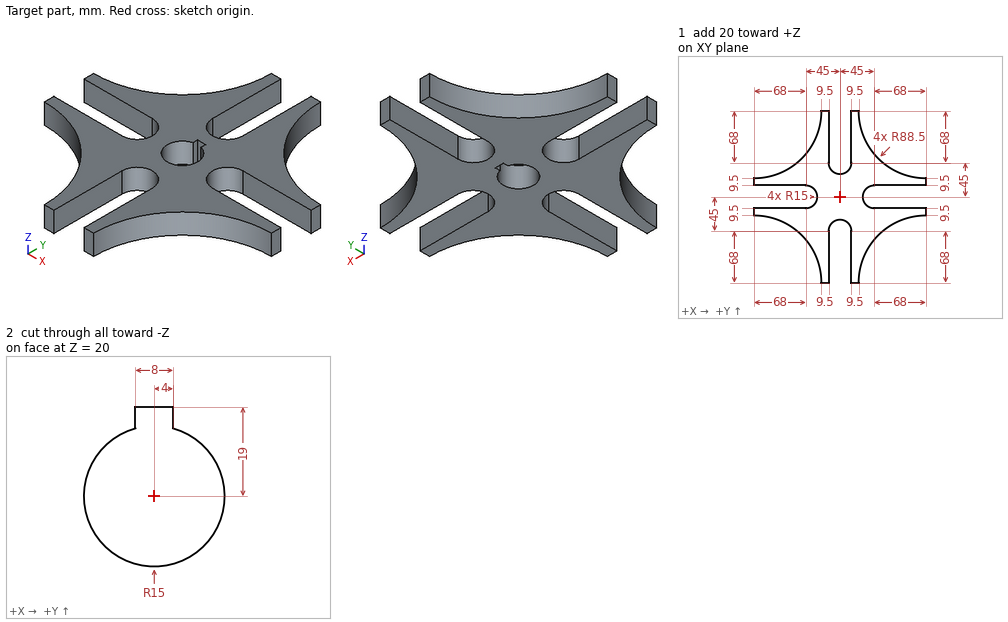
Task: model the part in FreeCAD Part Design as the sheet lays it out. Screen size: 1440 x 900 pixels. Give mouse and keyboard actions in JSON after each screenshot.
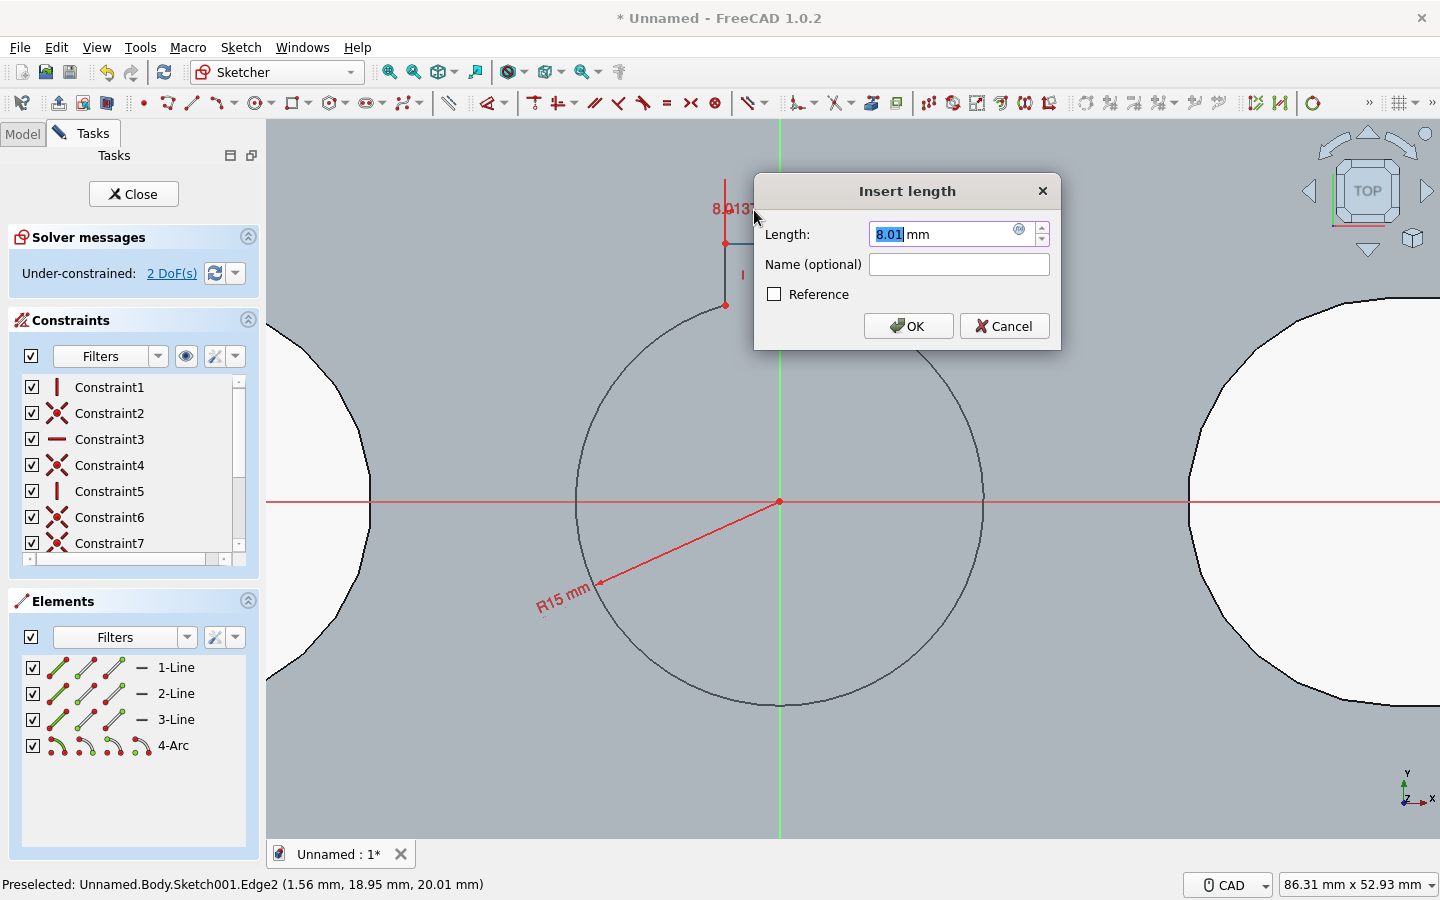
{"action": "type", "text": "8"}
{"action": "key", "text": "Return"}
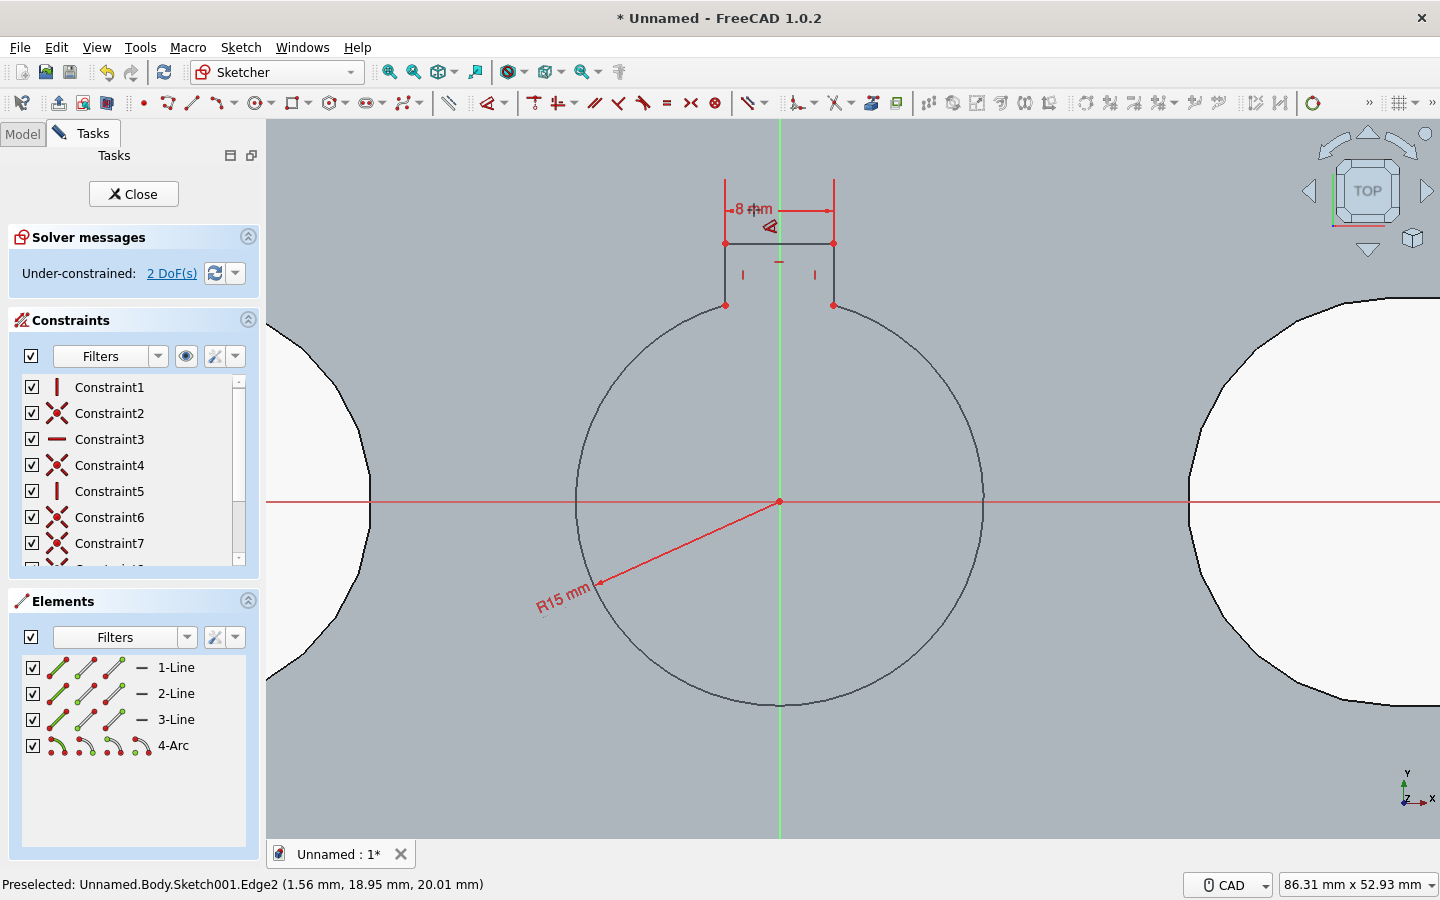
{"action": "left_click", "coordinate": [834, 305]}
{"action": "left_click", "coordinate": [807, 271]}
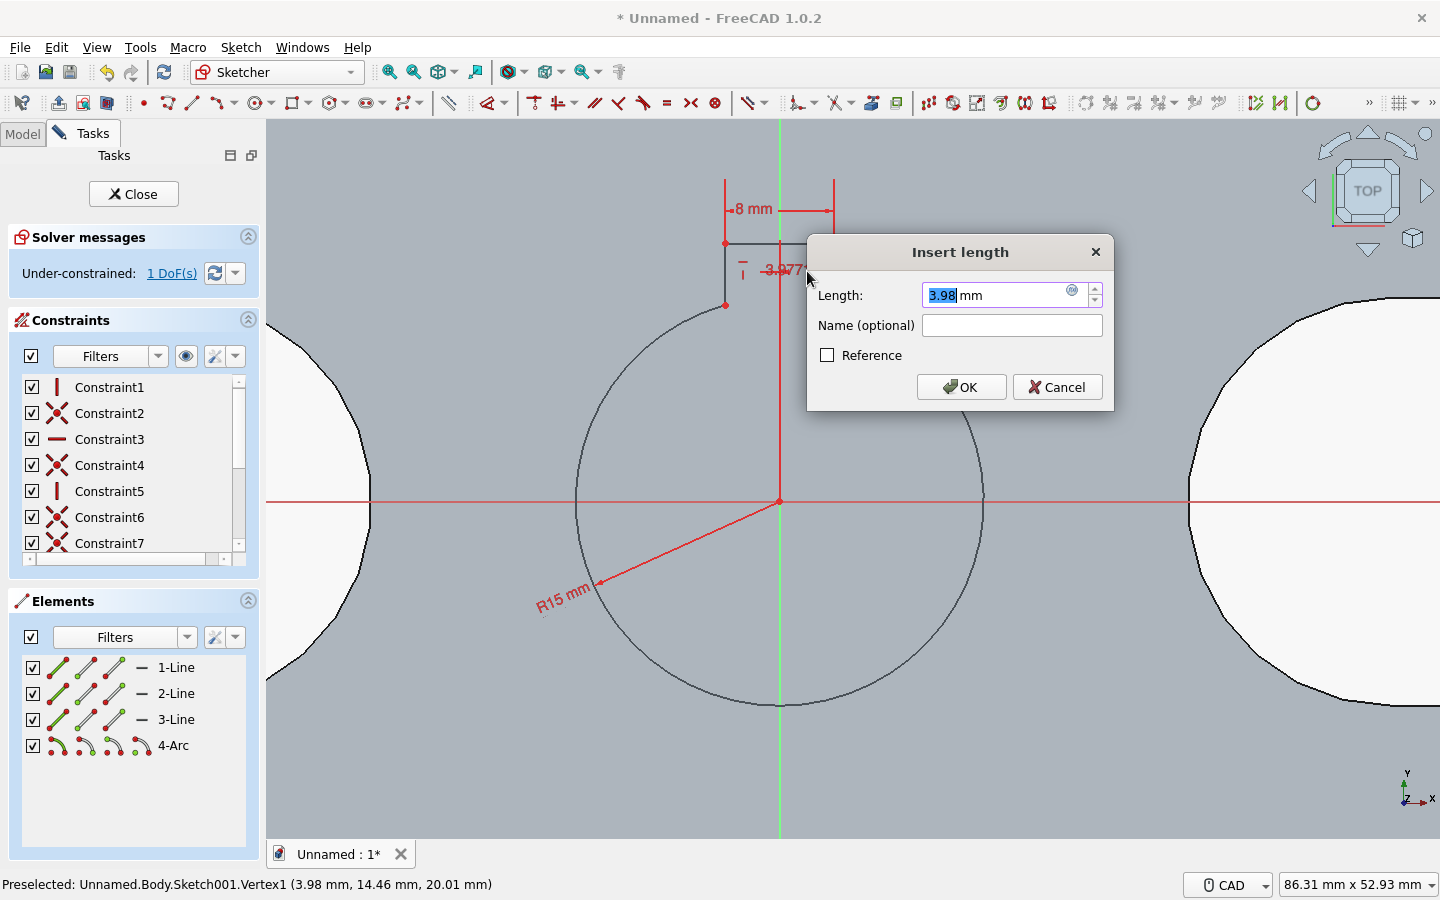
{"action": "type", "text": "4"}
{"action": "key", "text": "Return"}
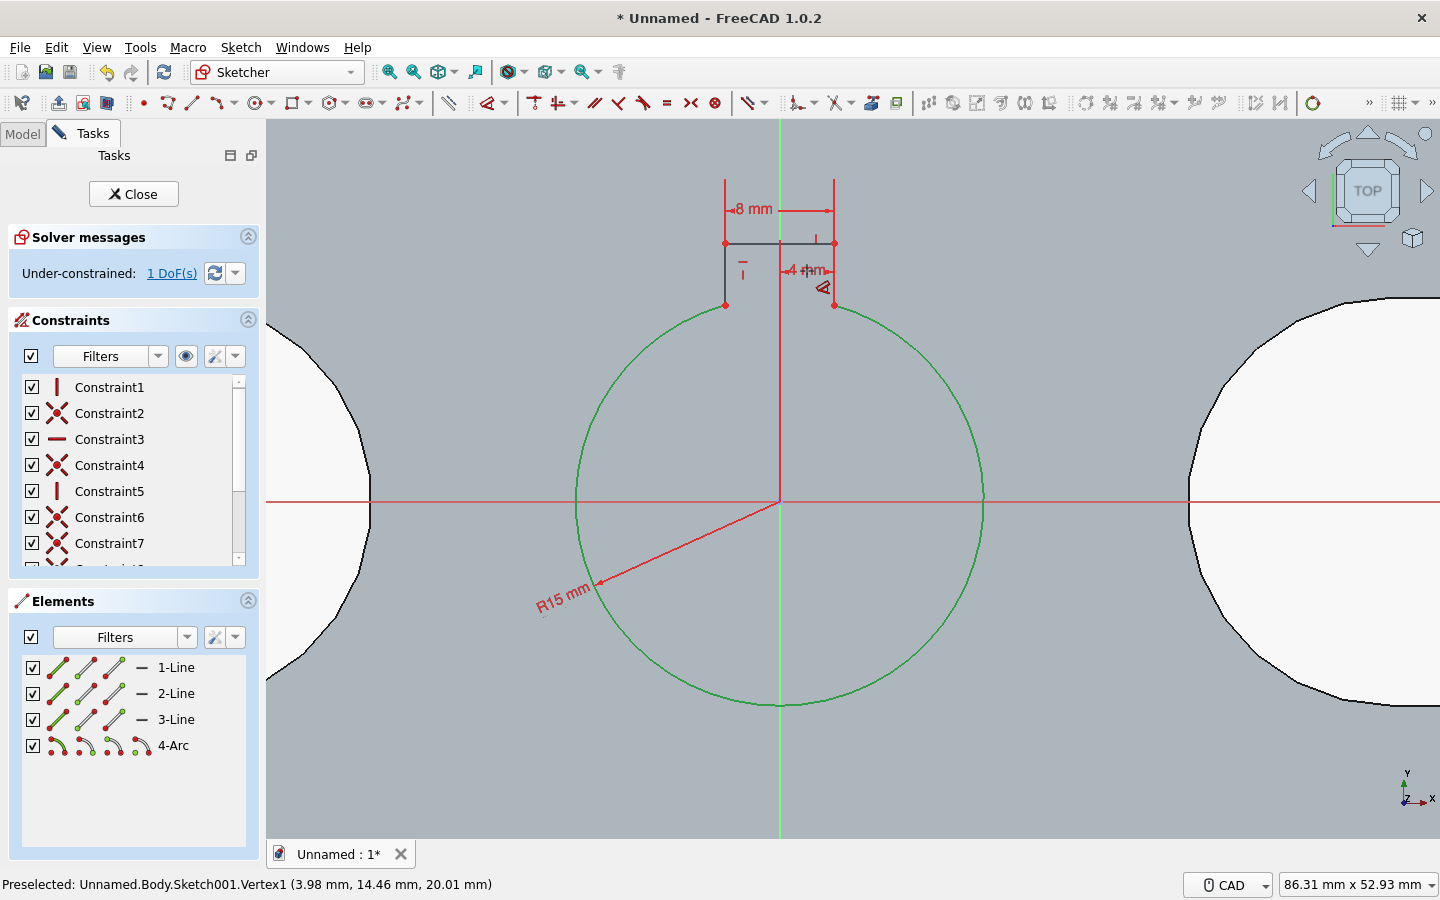
{"action": "left_click", "coordinate": [834, 244]}
{"action": "left_click", "coordinate": [868, 373]}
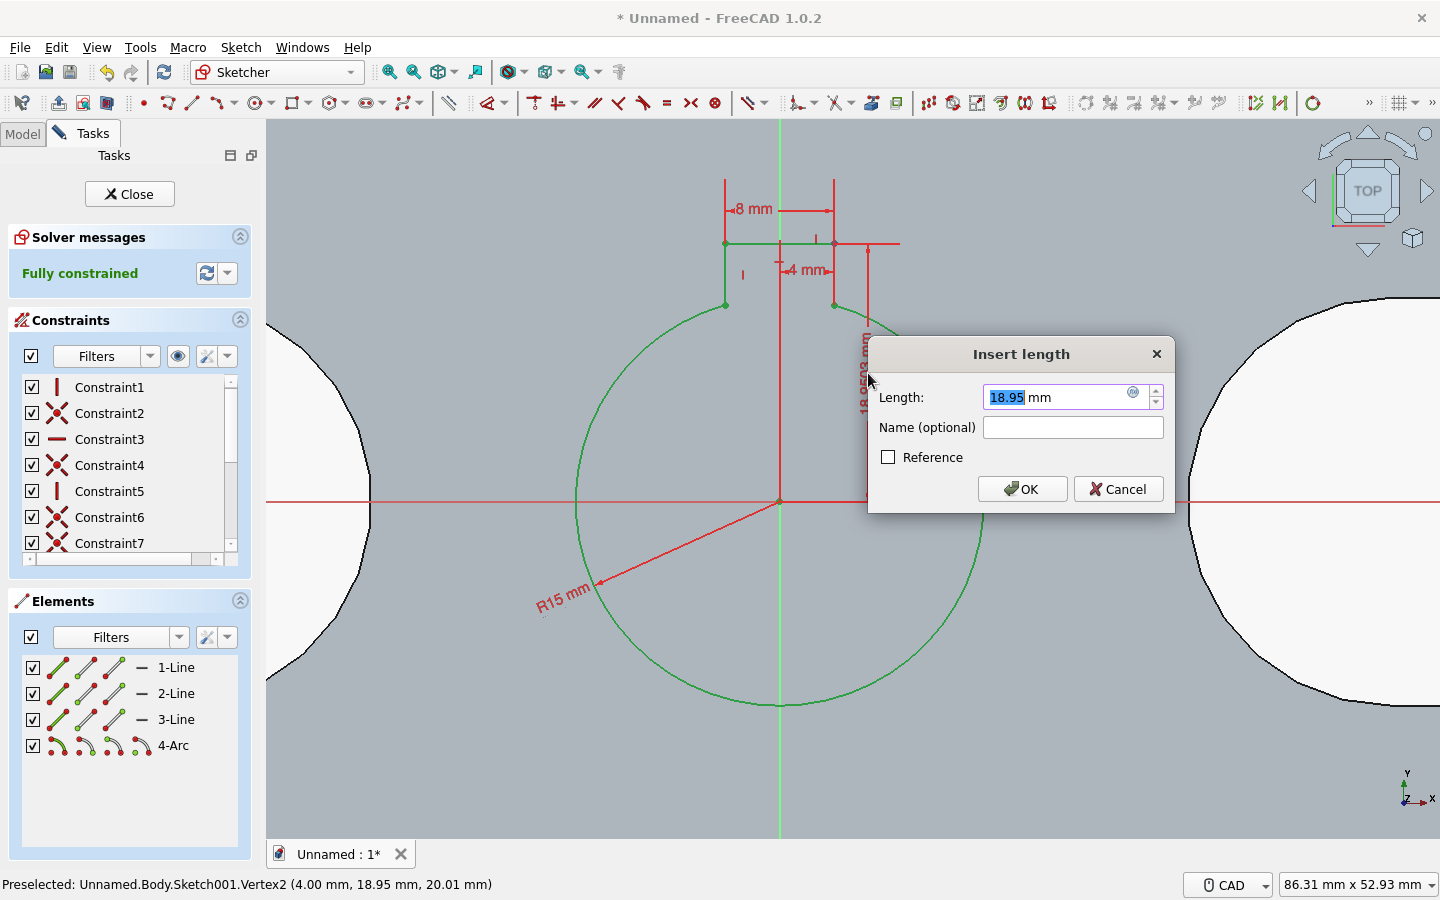
{"action": "type", "text": "19"}
{"action": "key", "text": "Return"}
{"action": "key", "text": "Escape"}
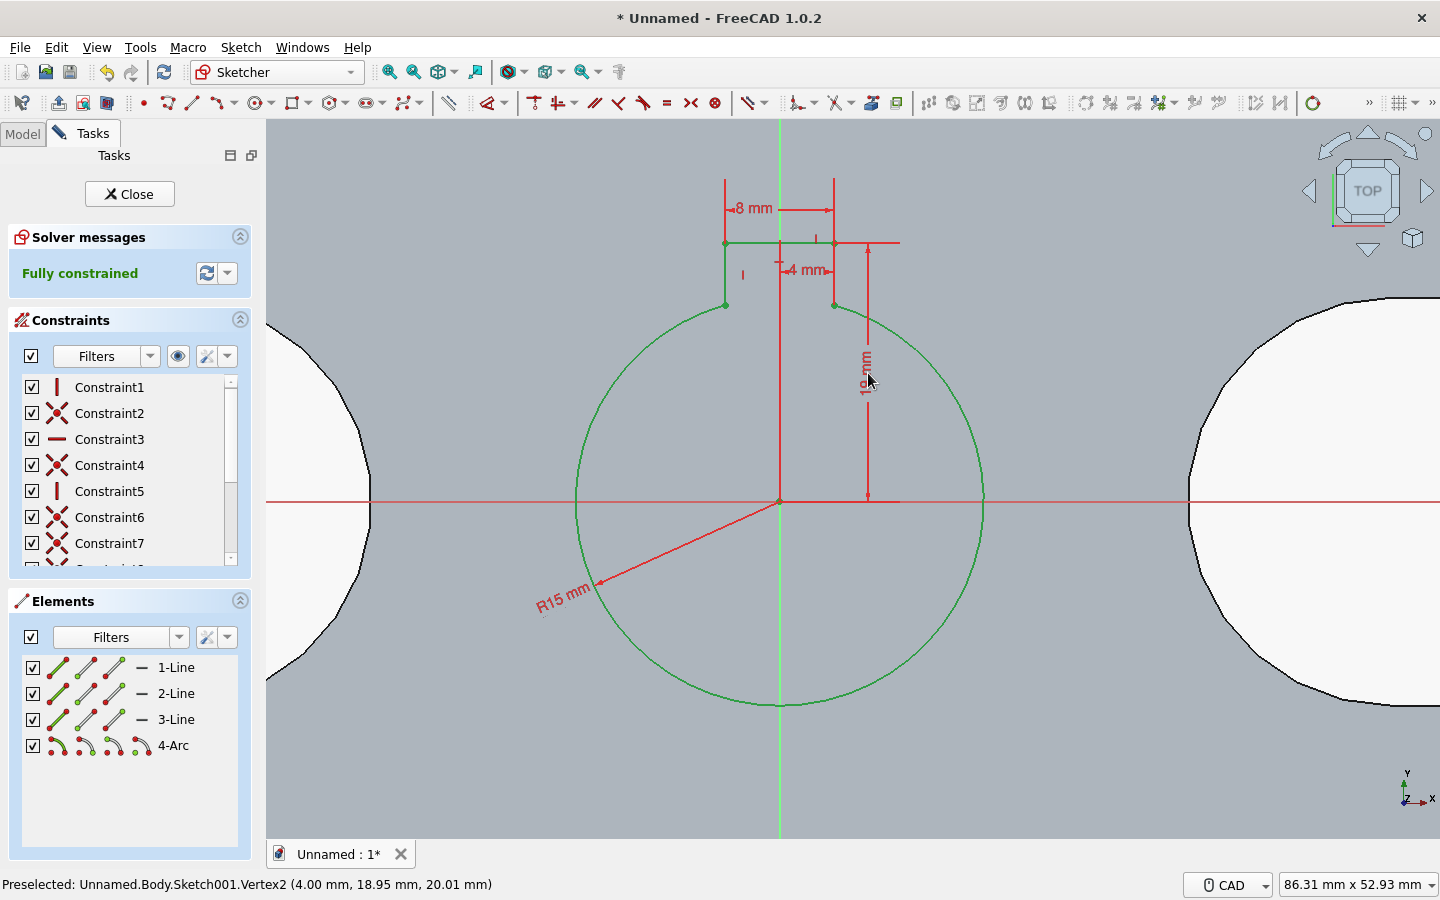
{"action": "left_click", "coordinate": [130, 194]}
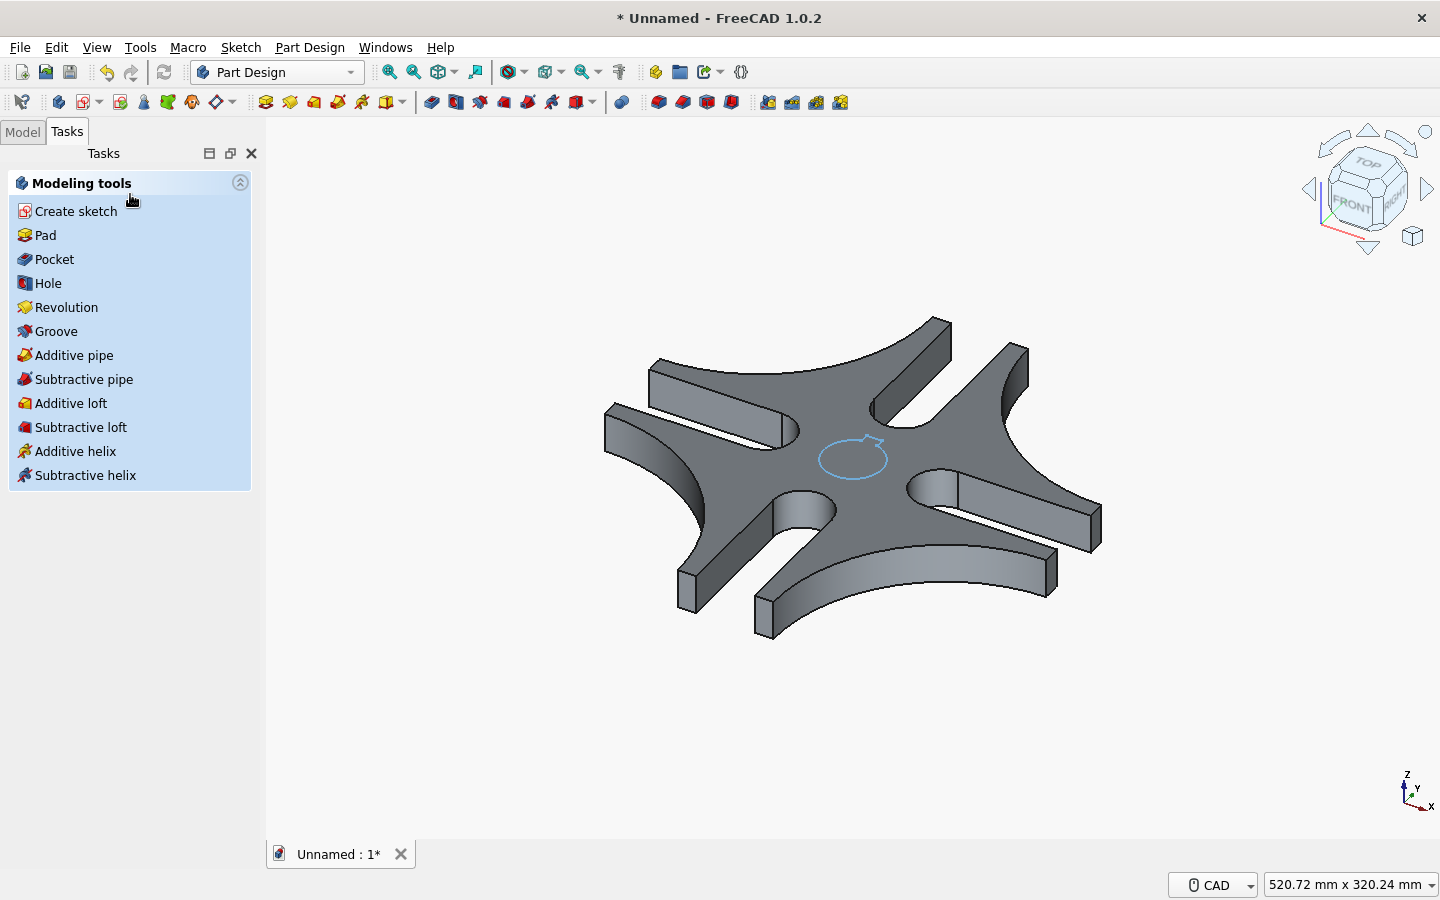
{"action": "left_click", "coordinate": [432, 102]}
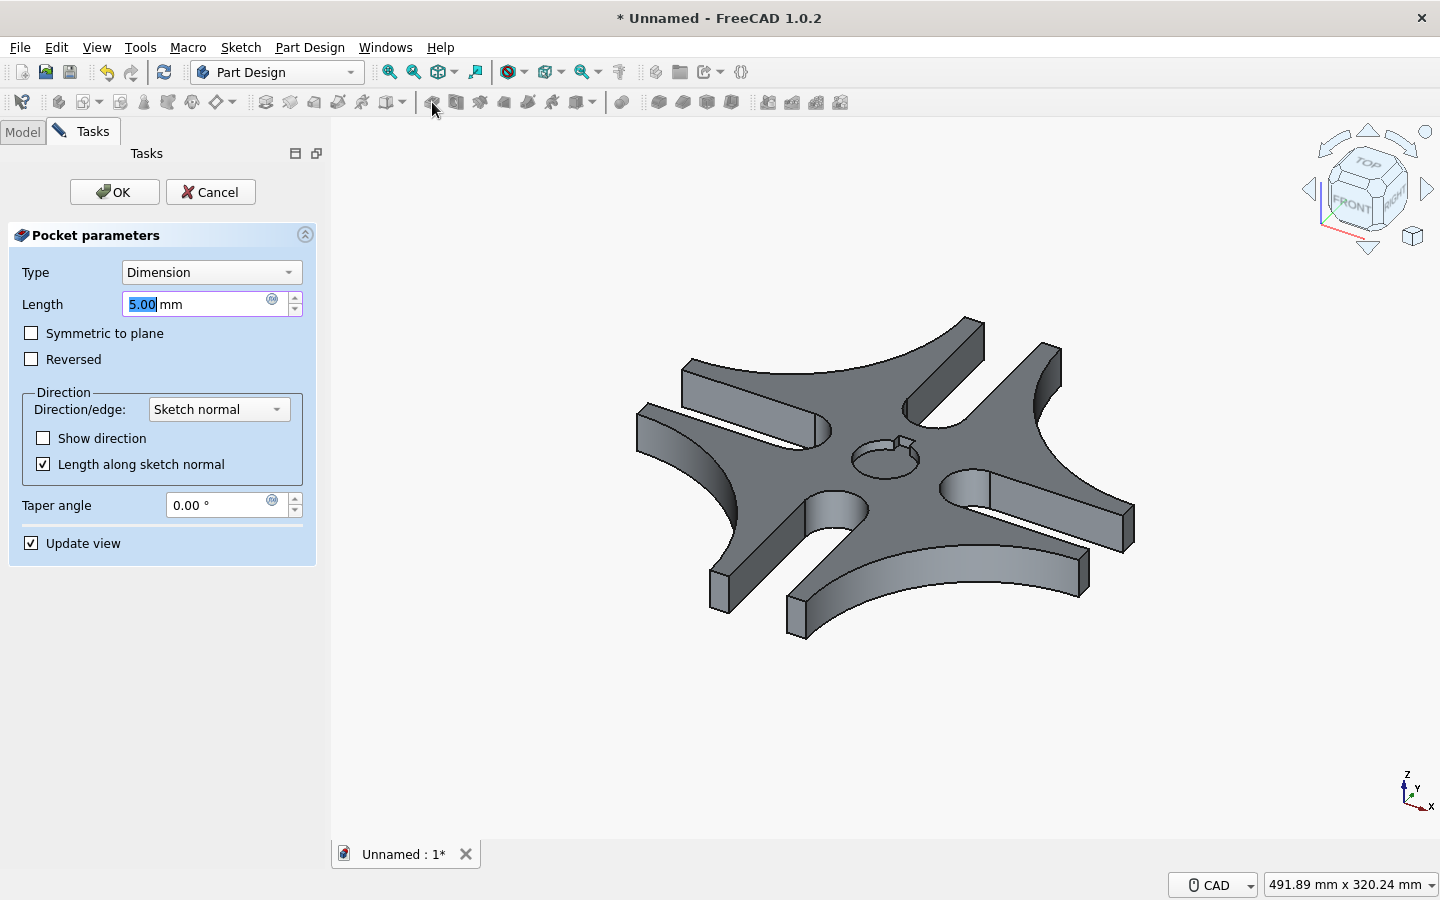
{"action": "left_click", "coordinate": [212, 272]}